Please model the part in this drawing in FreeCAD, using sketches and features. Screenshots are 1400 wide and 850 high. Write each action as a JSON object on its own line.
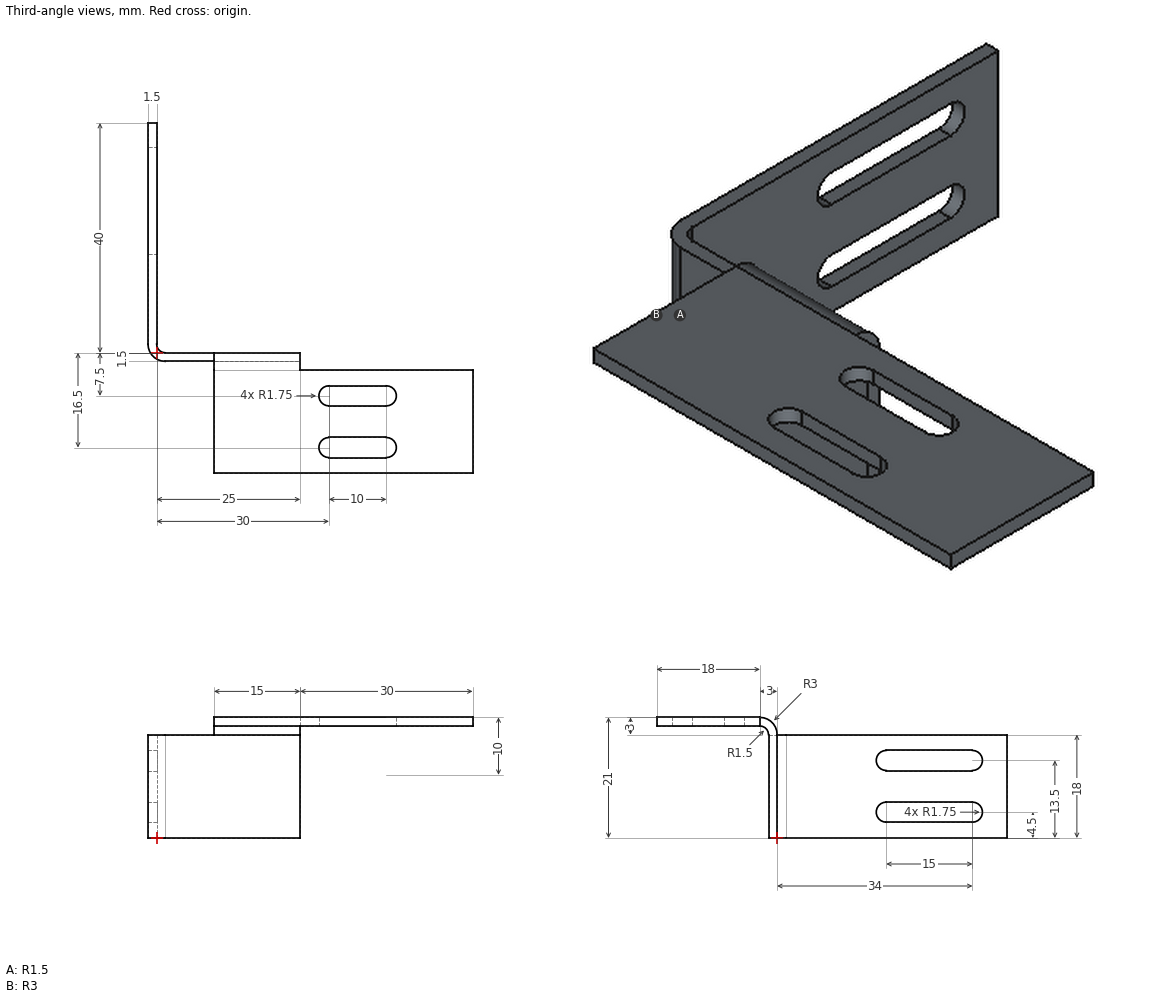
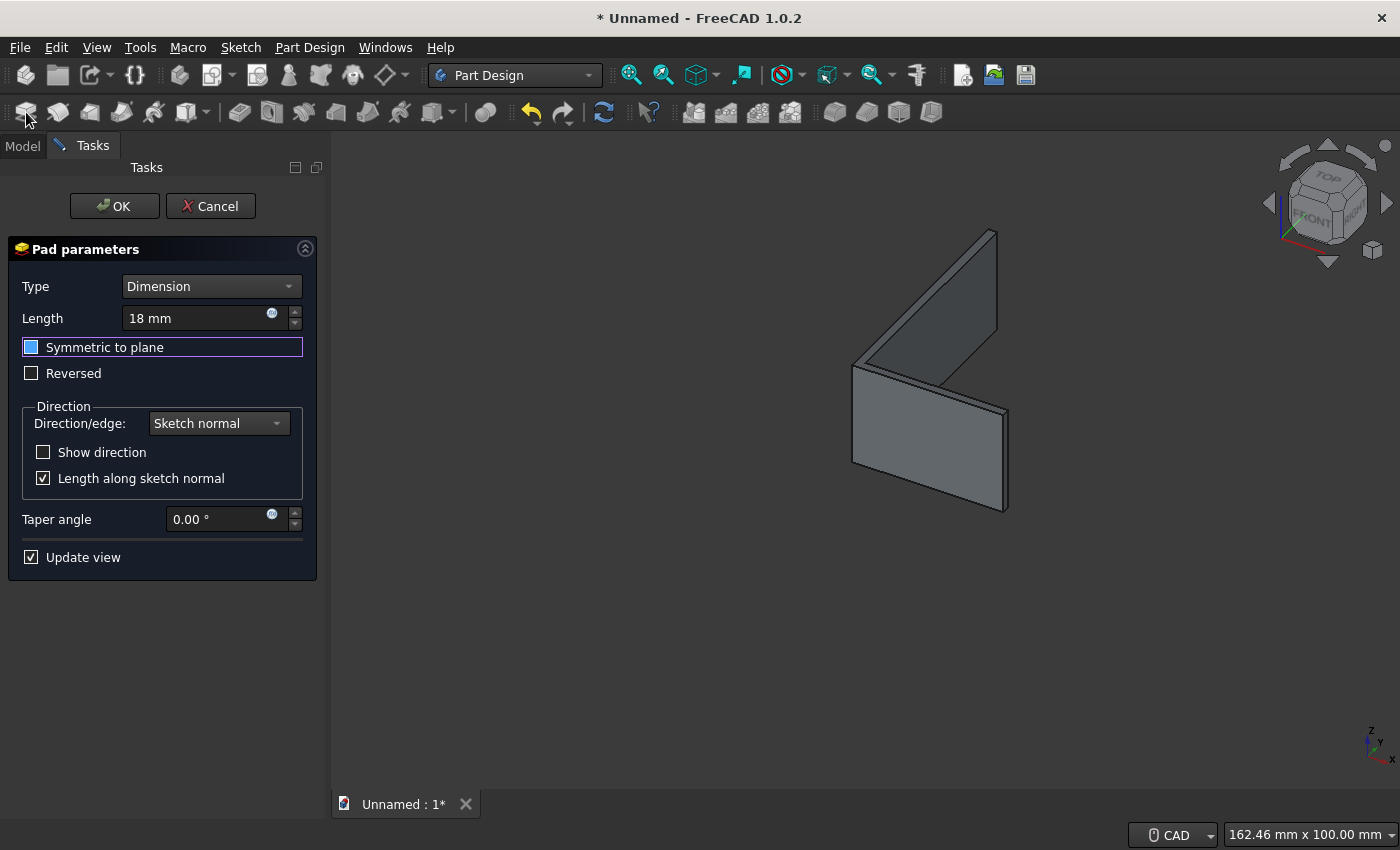
{"action": "left_click", "coordinate": [115, 206]}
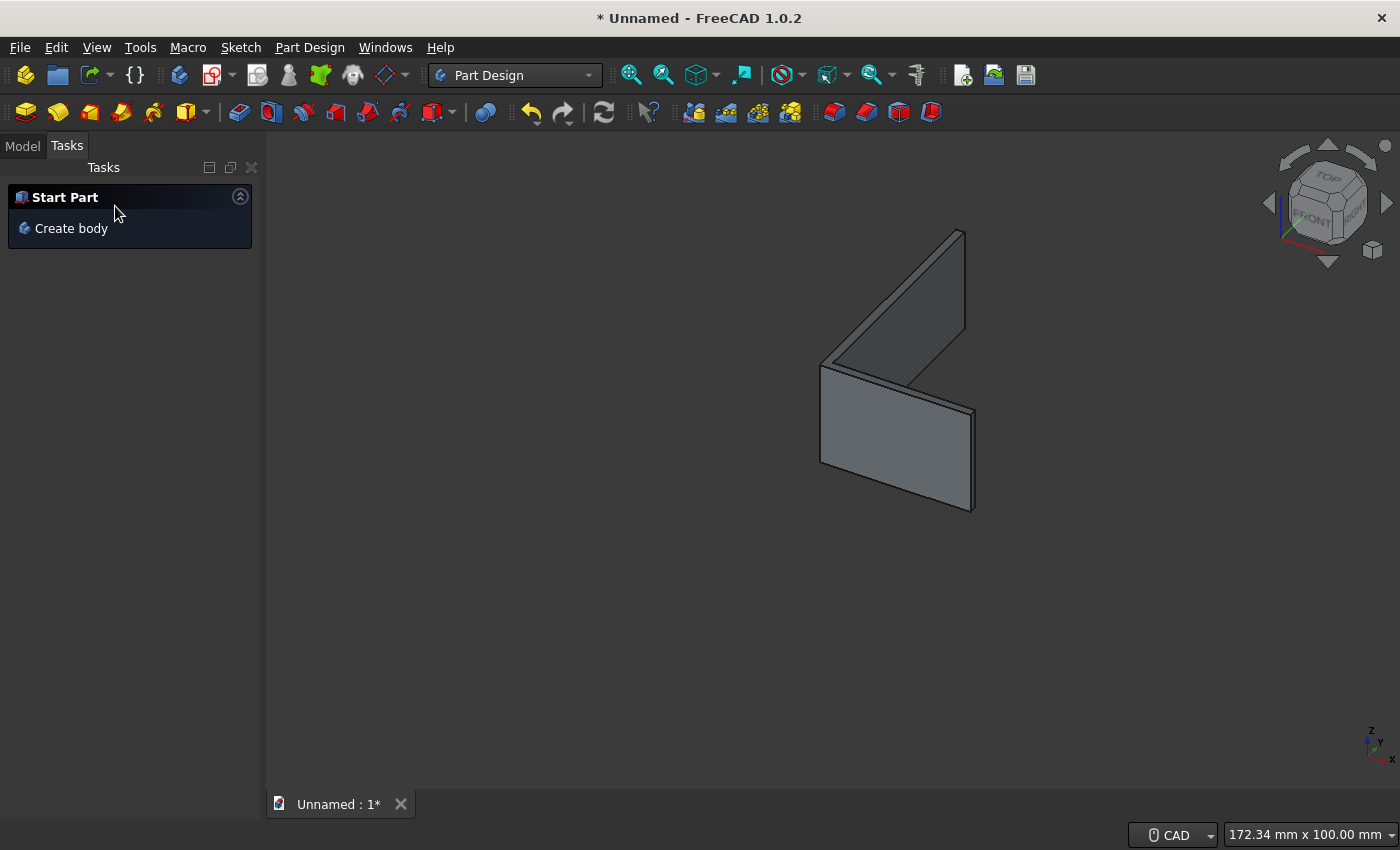
{"action": "key", "text": "v f"}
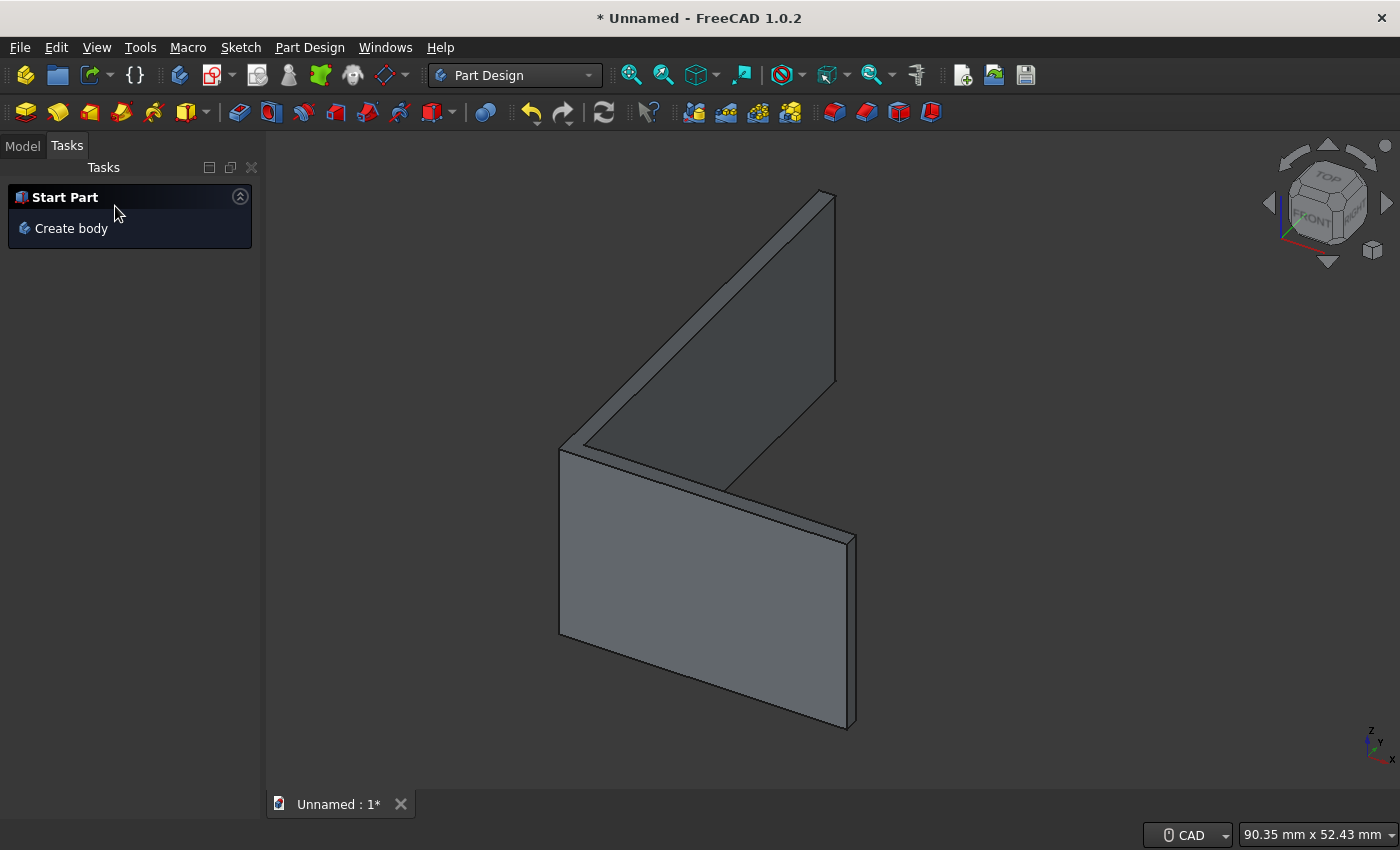
{"action": "key", "text": "0"}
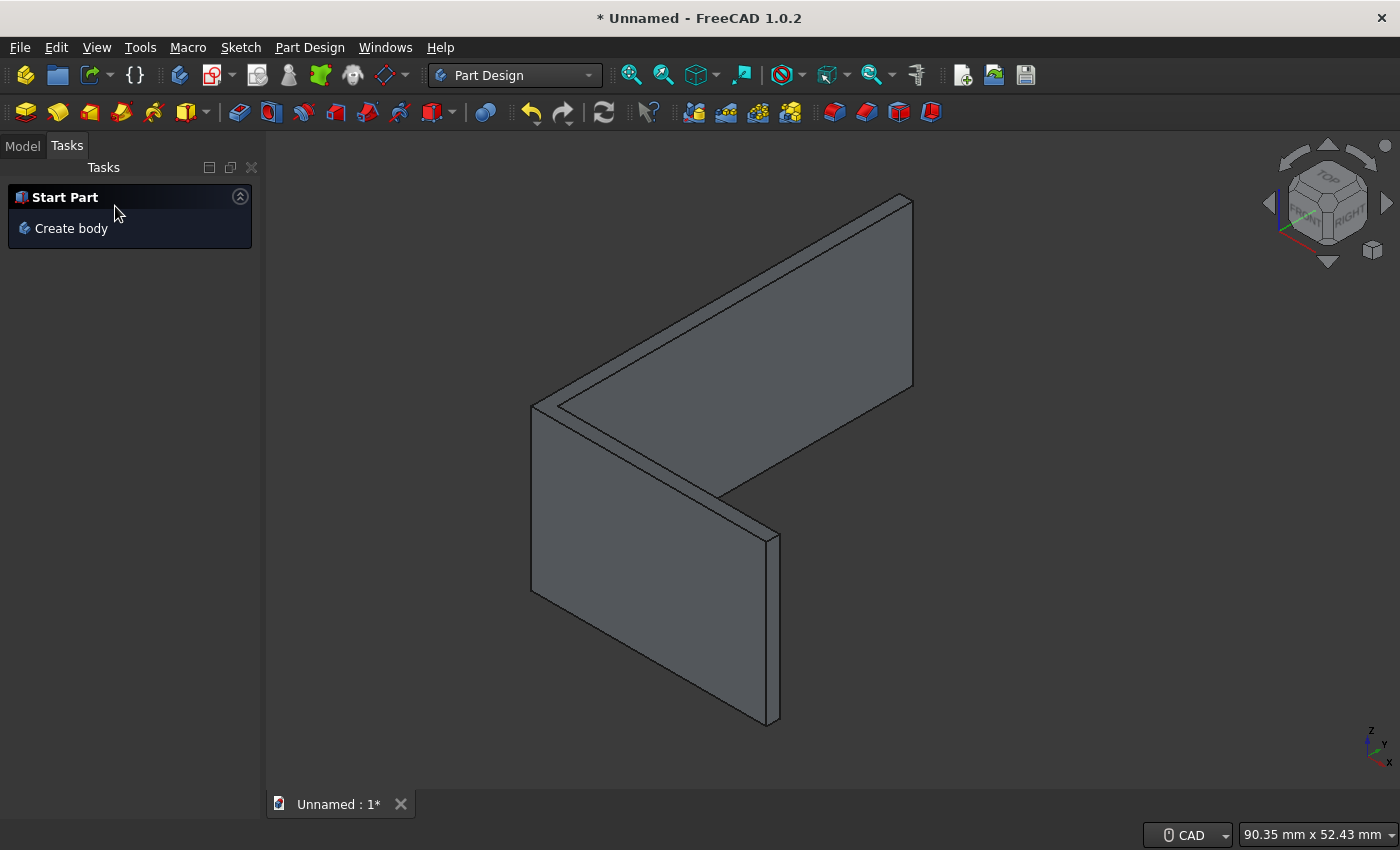
{"action": "key", "text": "2"}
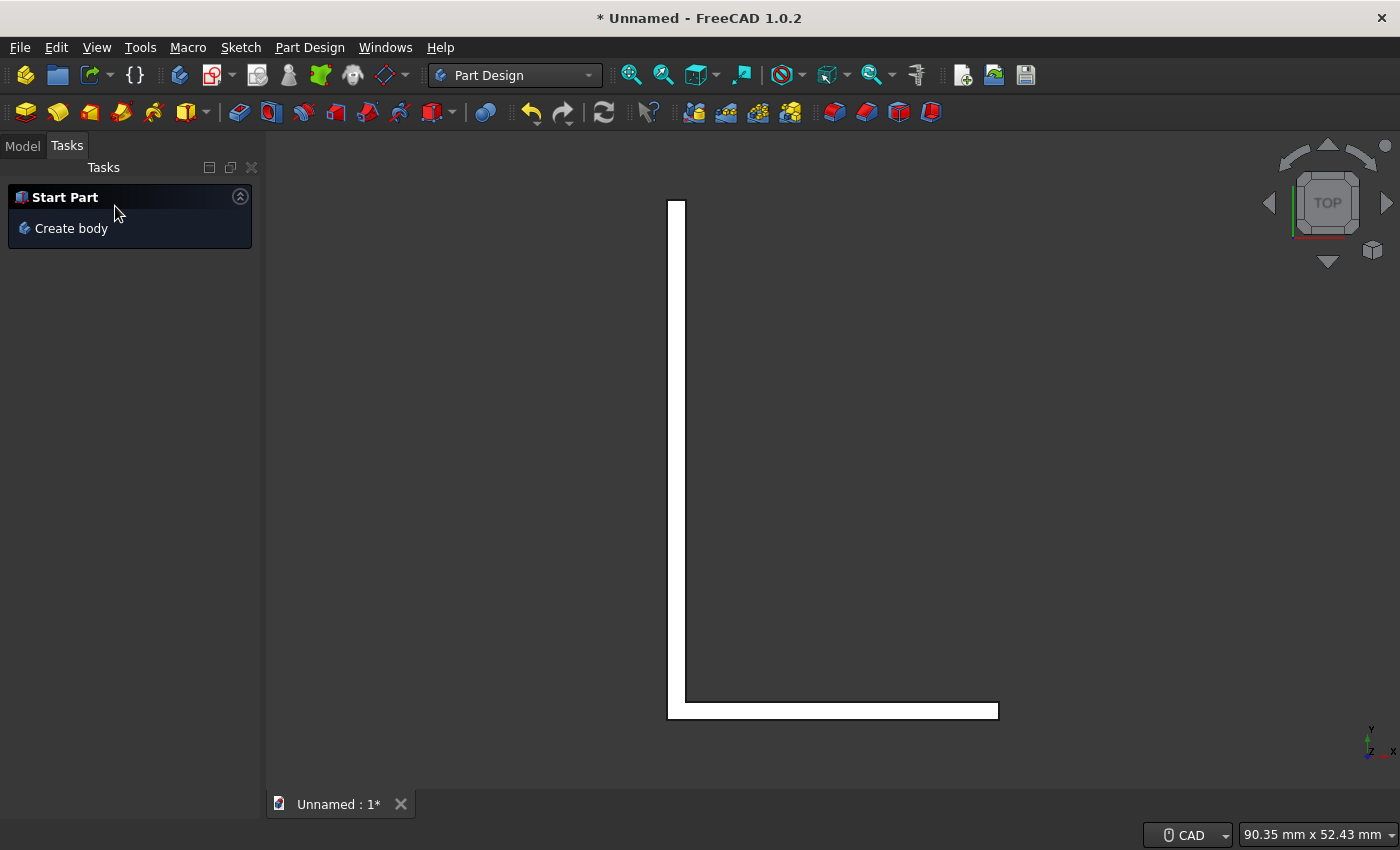
{"action": "key", "text": "1"}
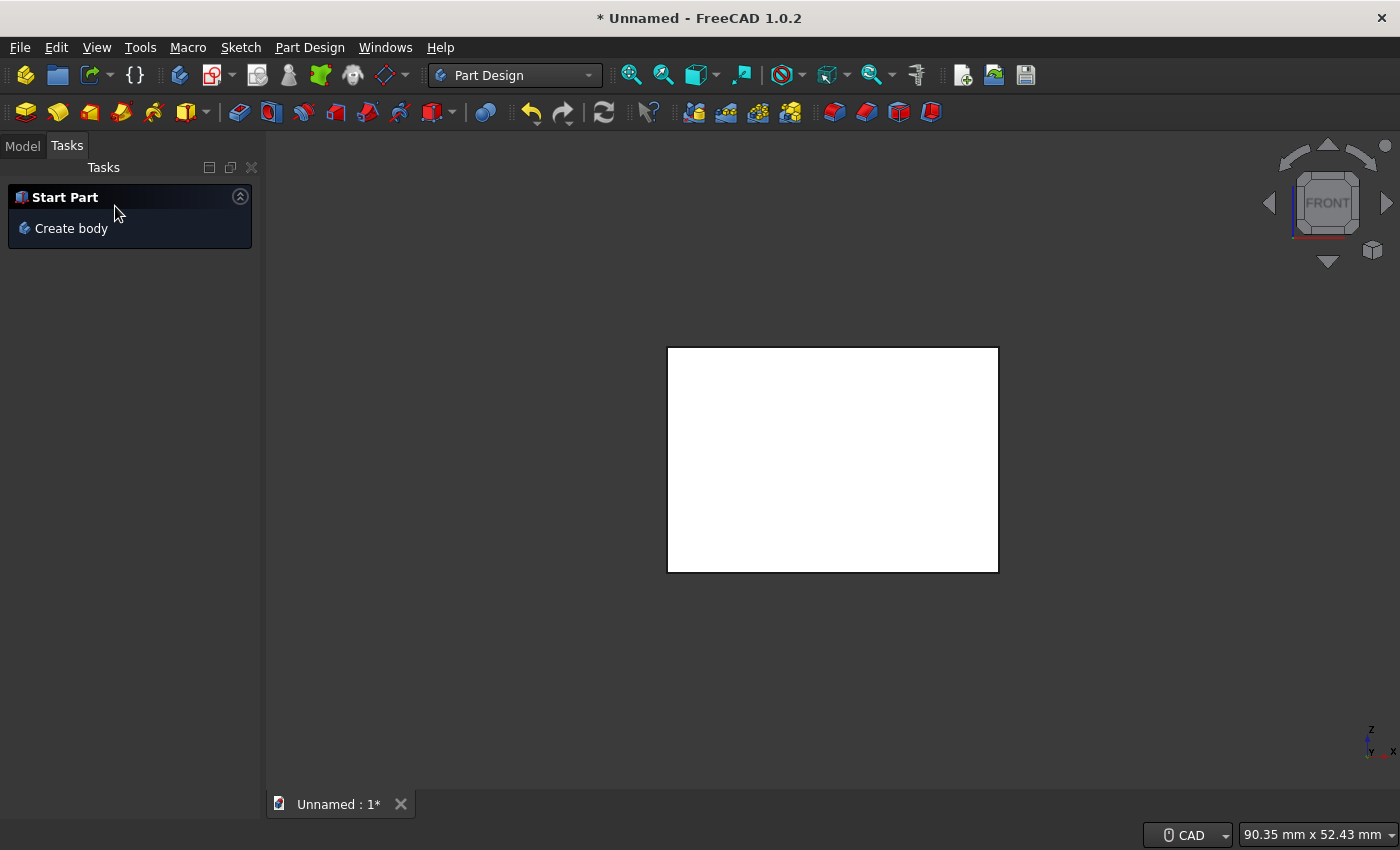
{"action": "key", "text": "v f"}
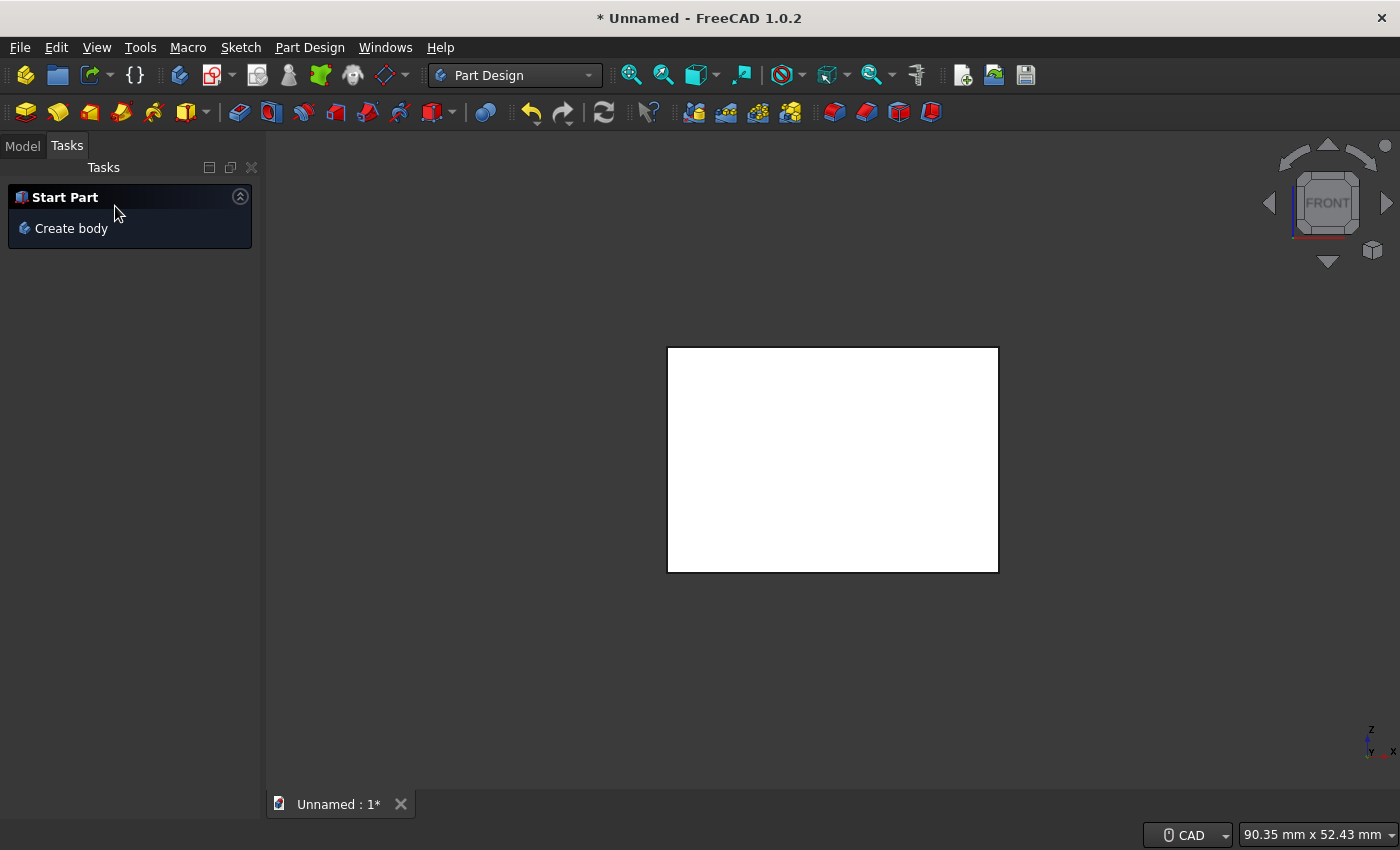
{"action": "key", "text": "3"}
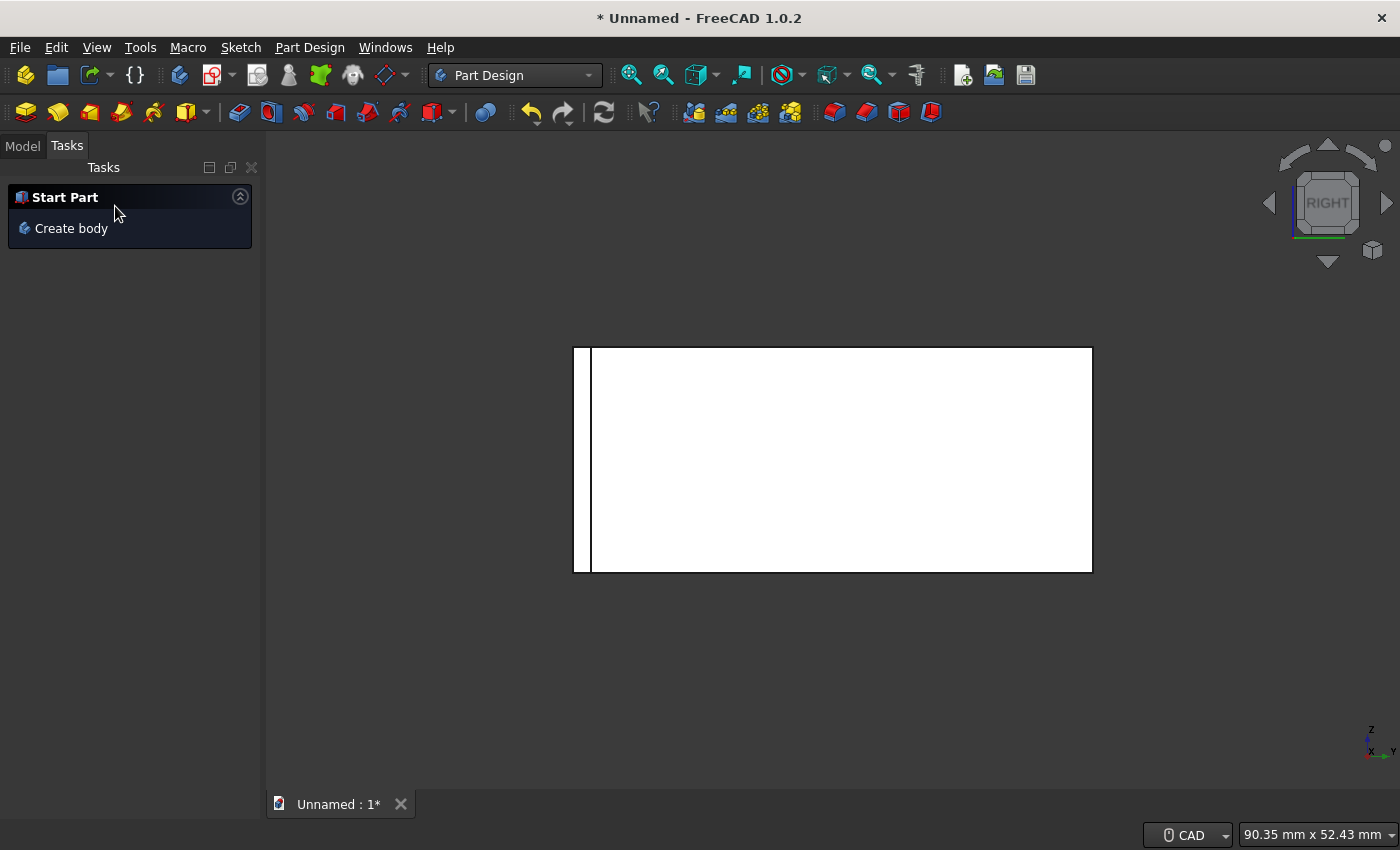
{"action": "key", "text": "5"}